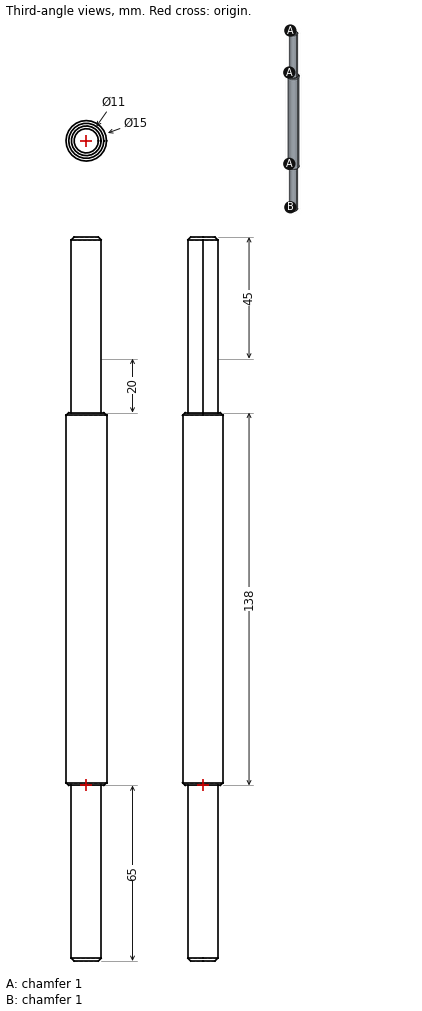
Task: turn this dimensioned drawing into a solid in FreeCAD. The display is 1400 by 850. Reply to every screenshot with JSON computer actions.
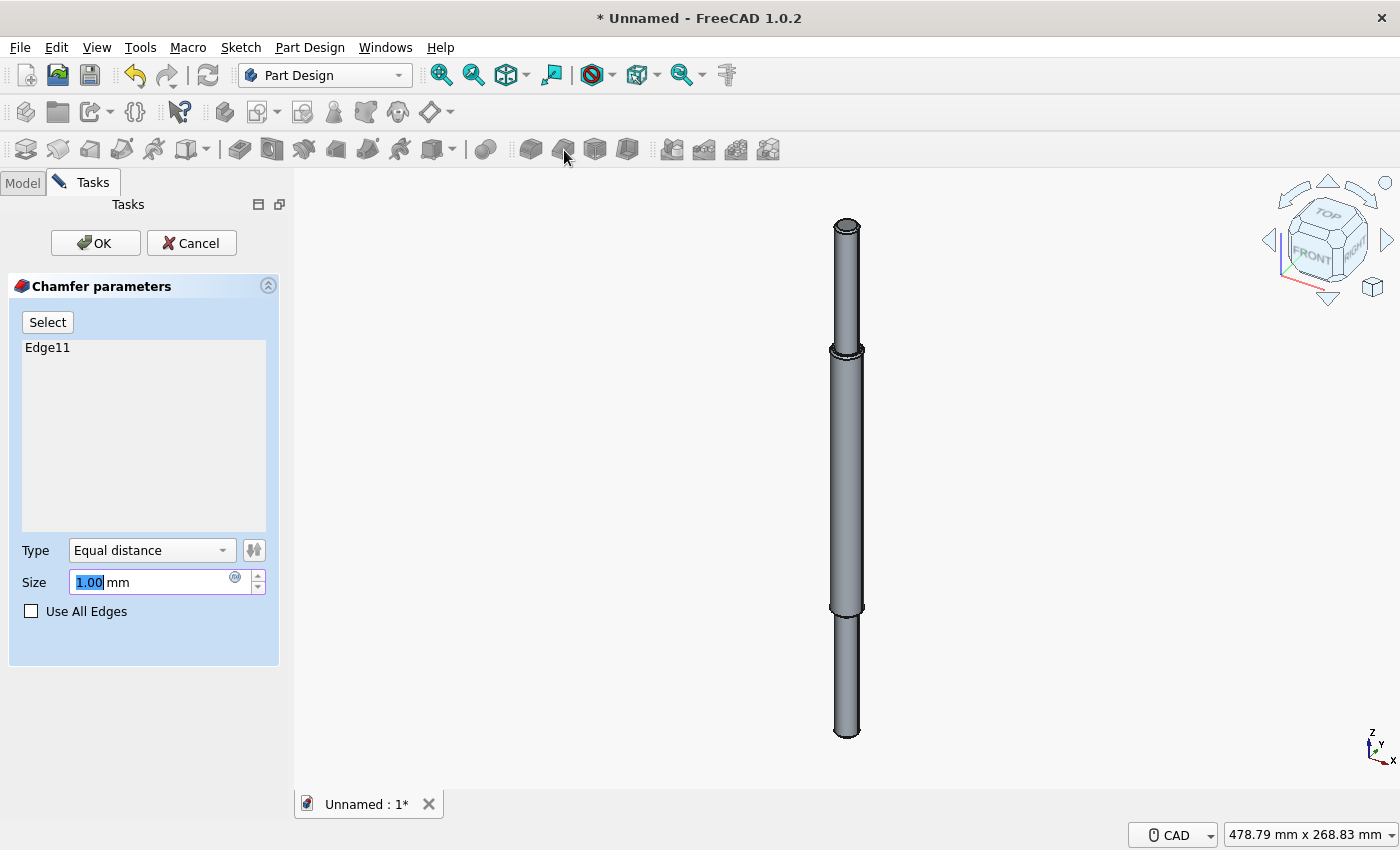
{"action": "type", "text": "1"}
{"action": "key", "text": "Tab"}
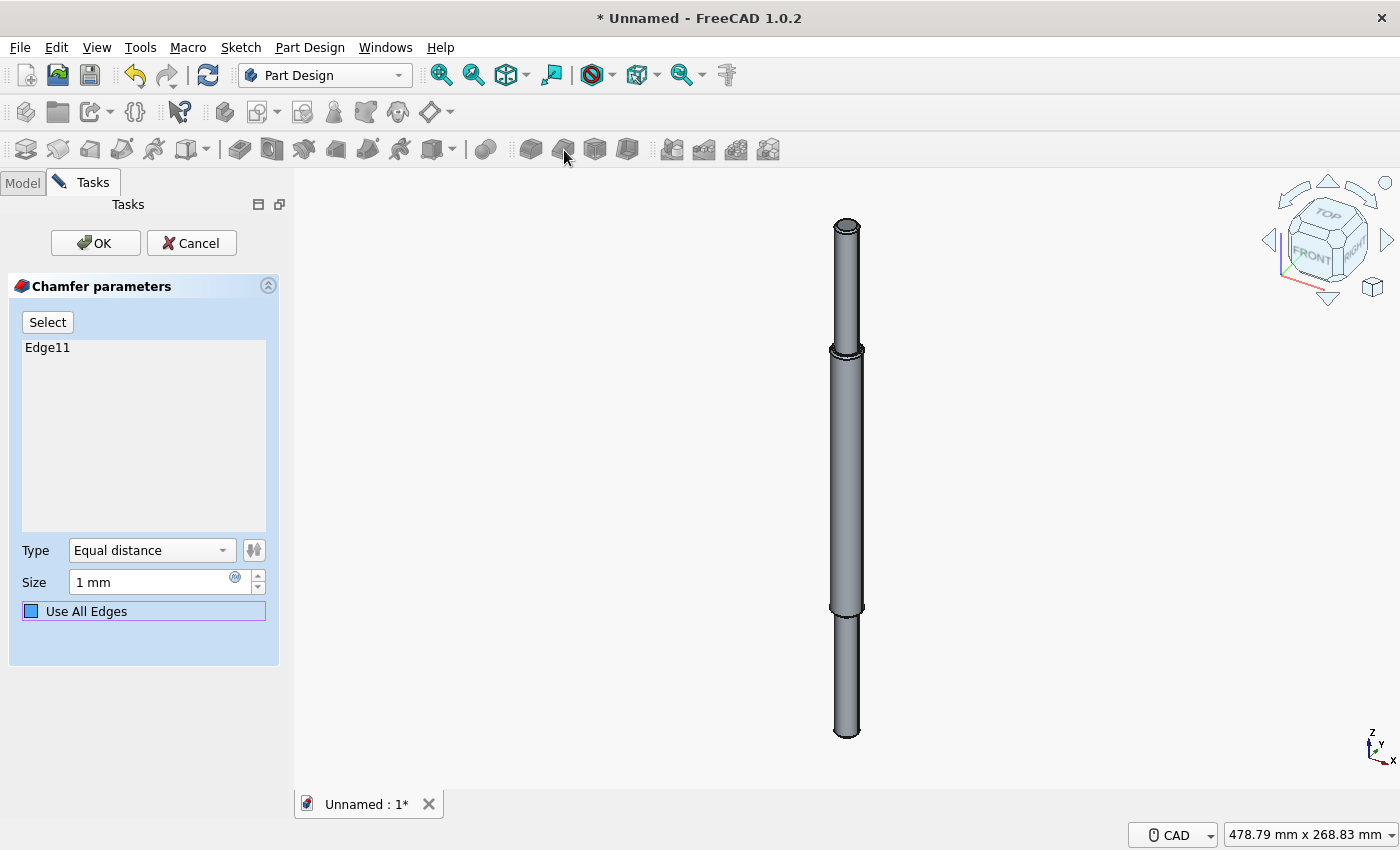
{"action": "left_click", "coordinate": [96, 243]}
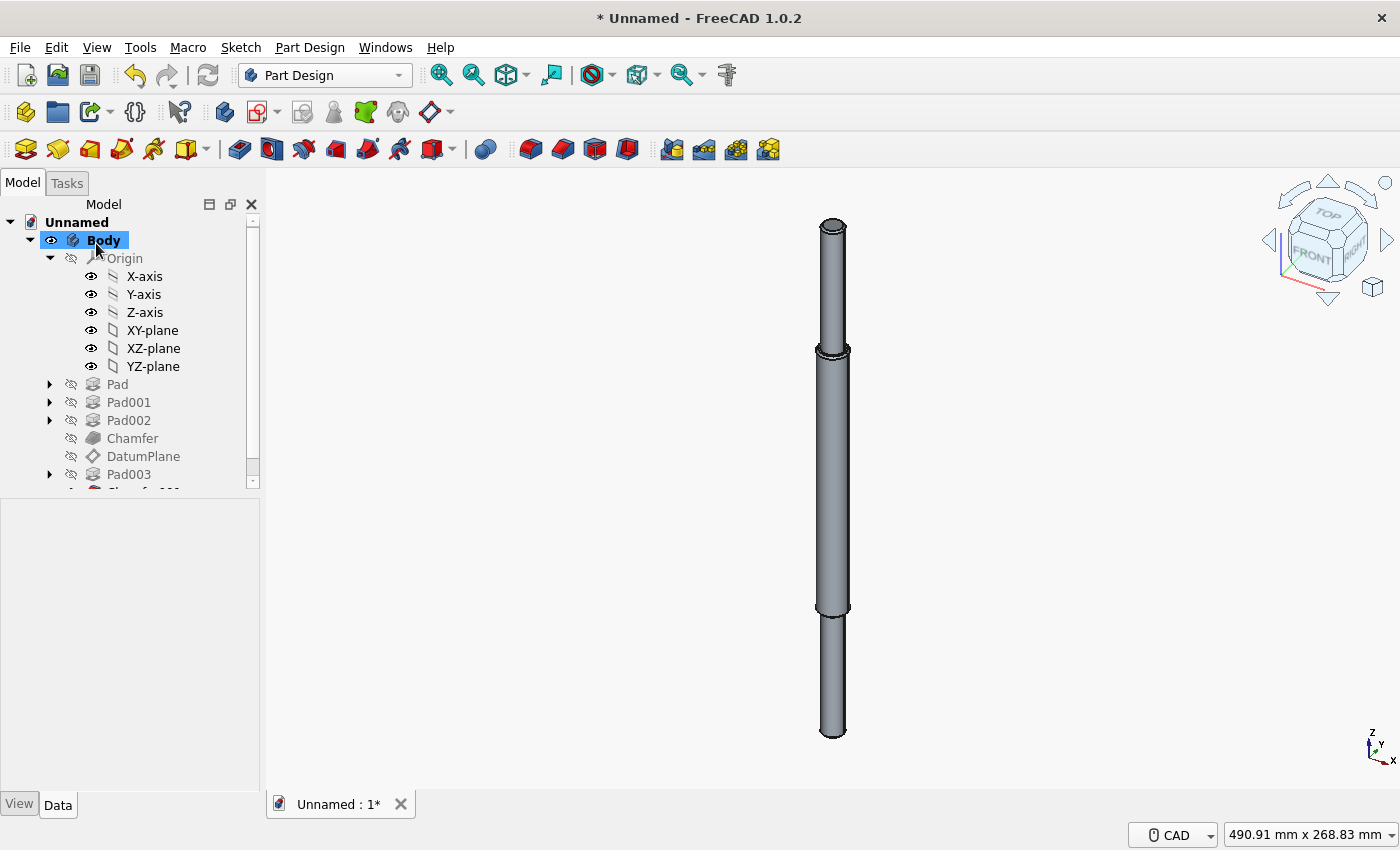
{"action": "key", "text": "0"}